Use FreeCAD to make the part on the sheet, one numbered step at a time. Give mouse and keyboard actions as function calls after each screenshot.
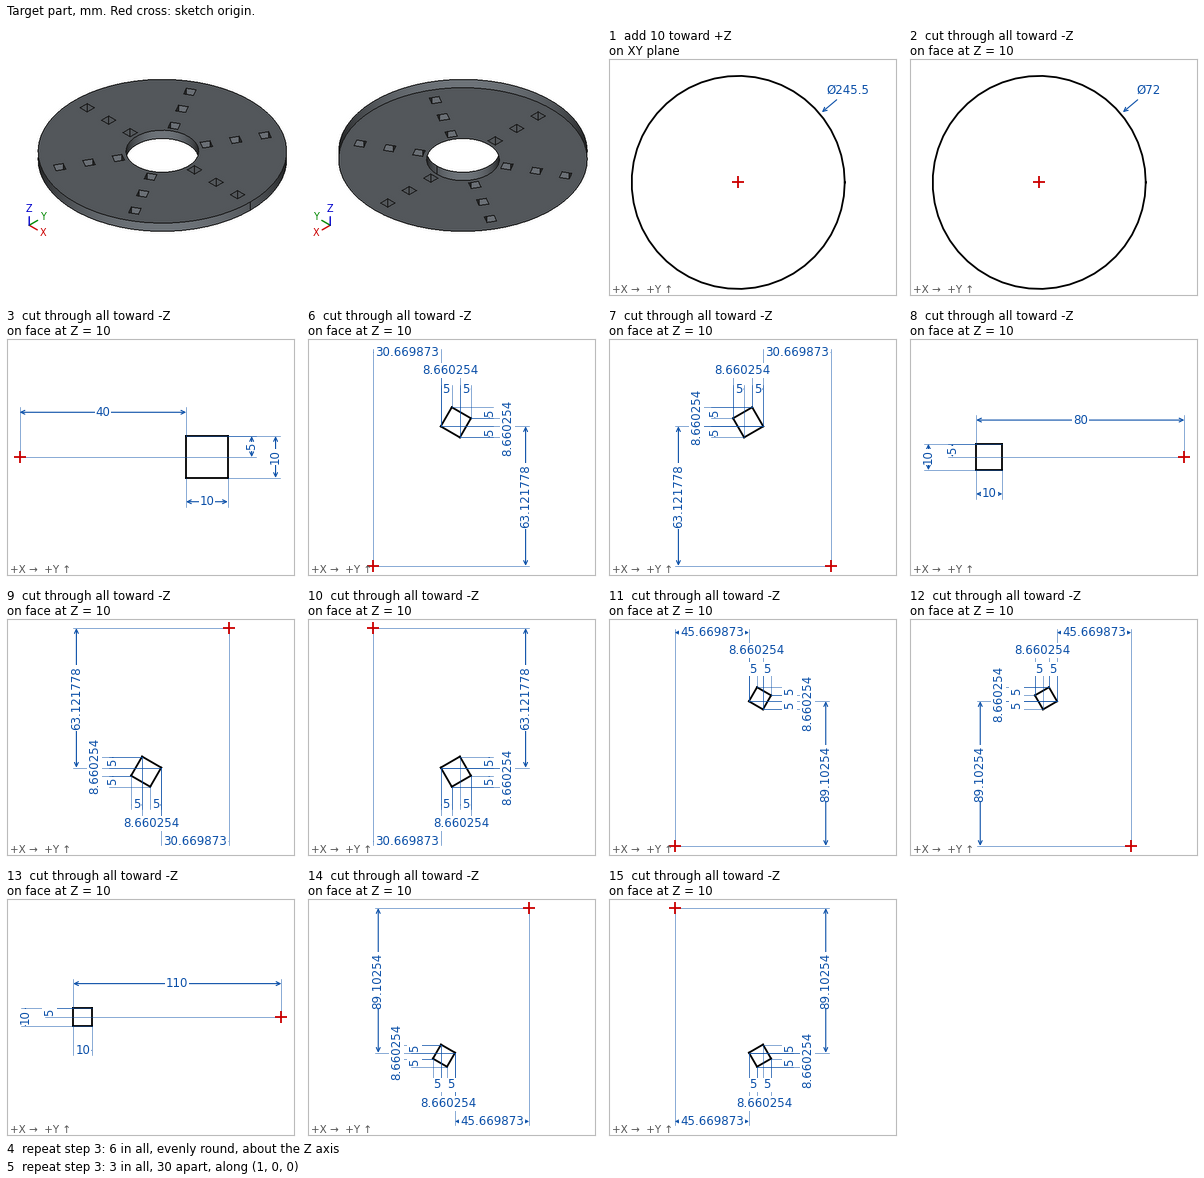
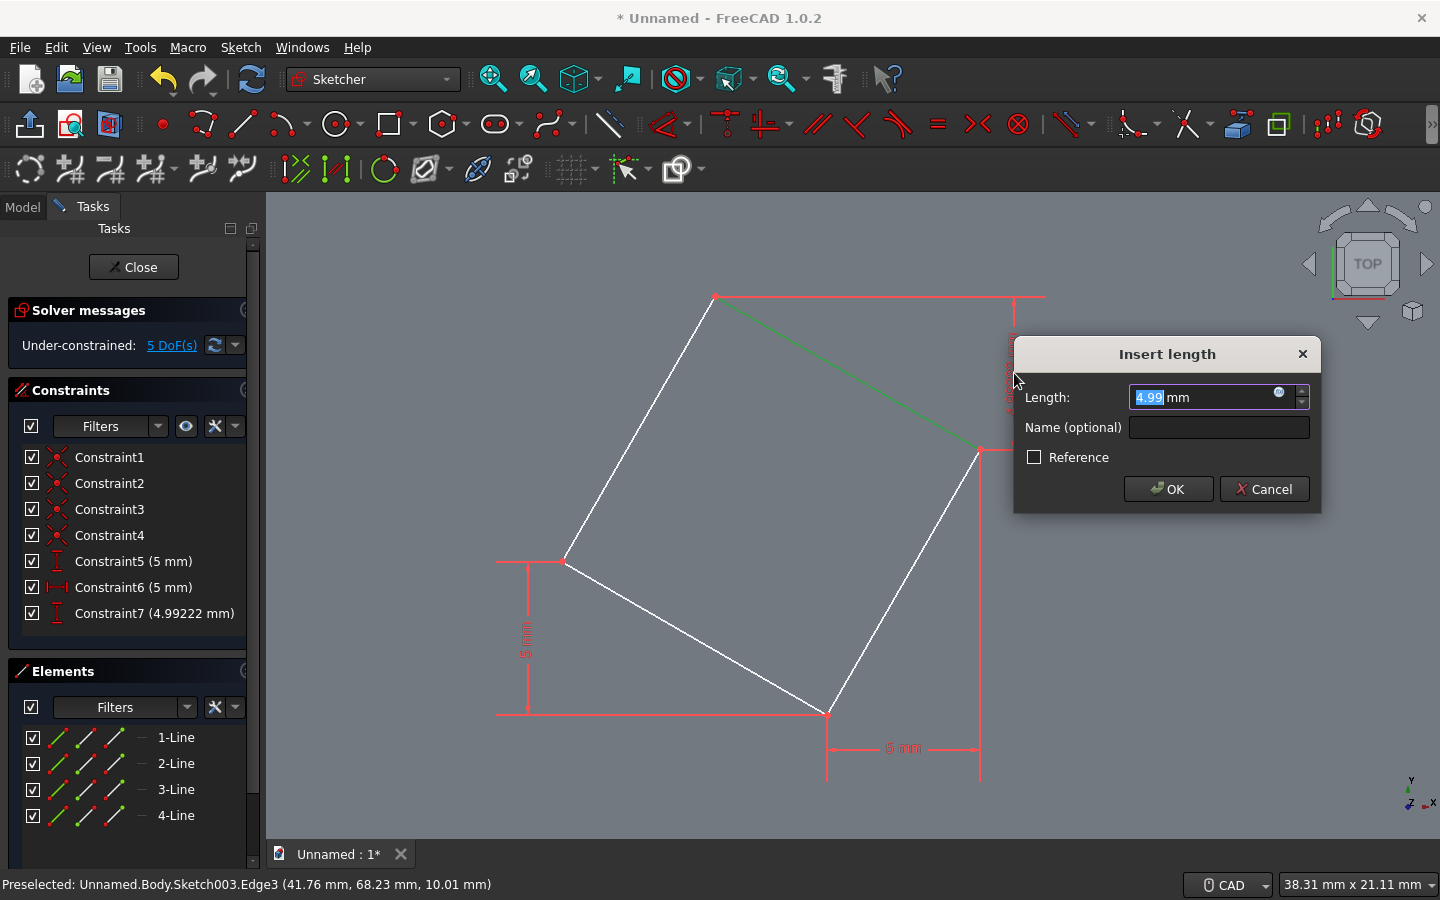
text(5)
key(Return)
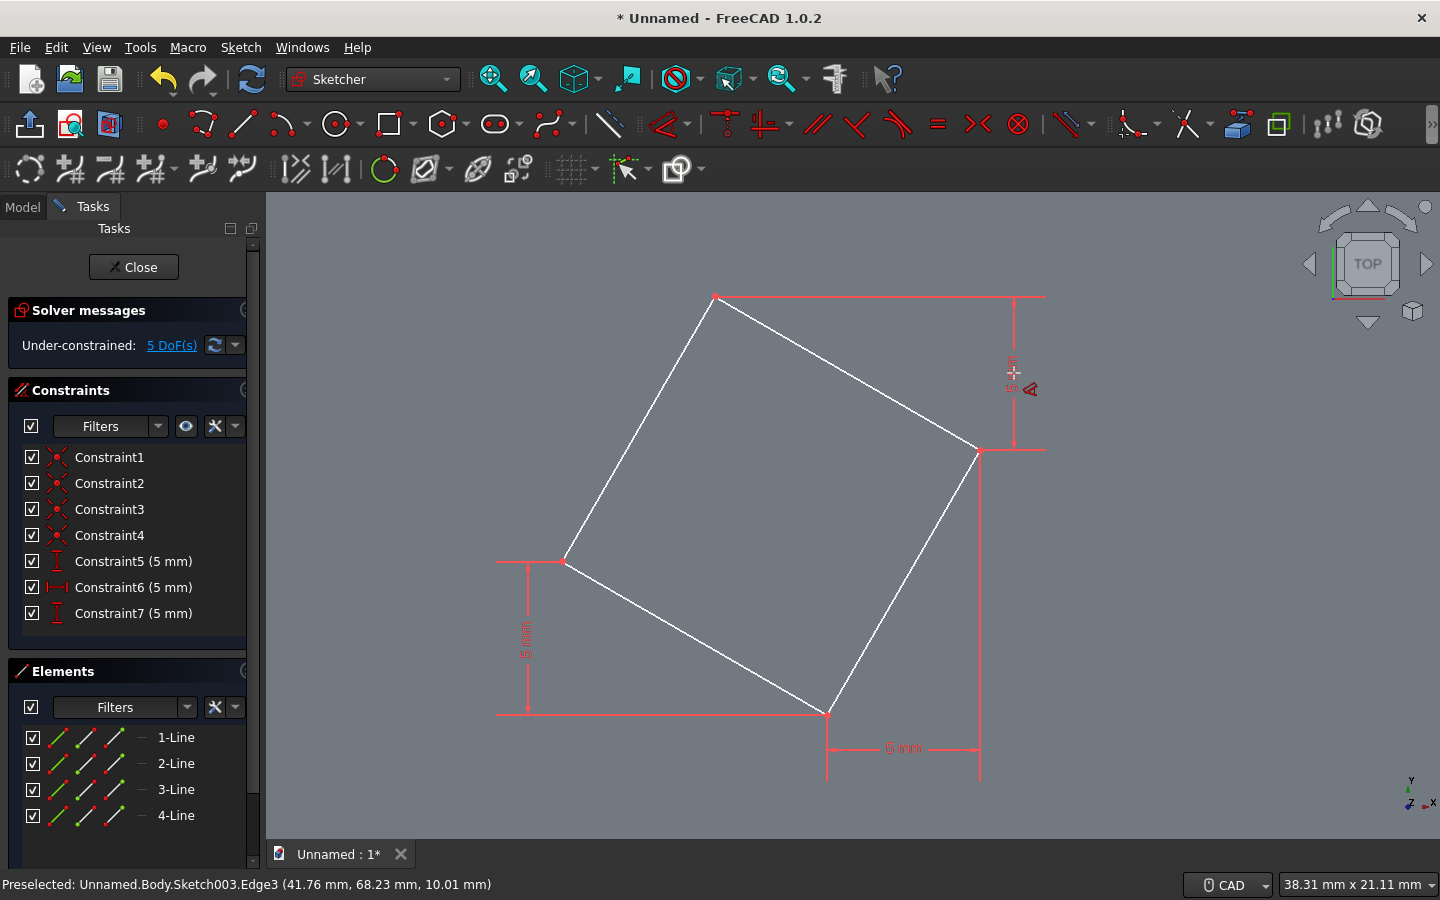
click(669, 376)
click(639, 263)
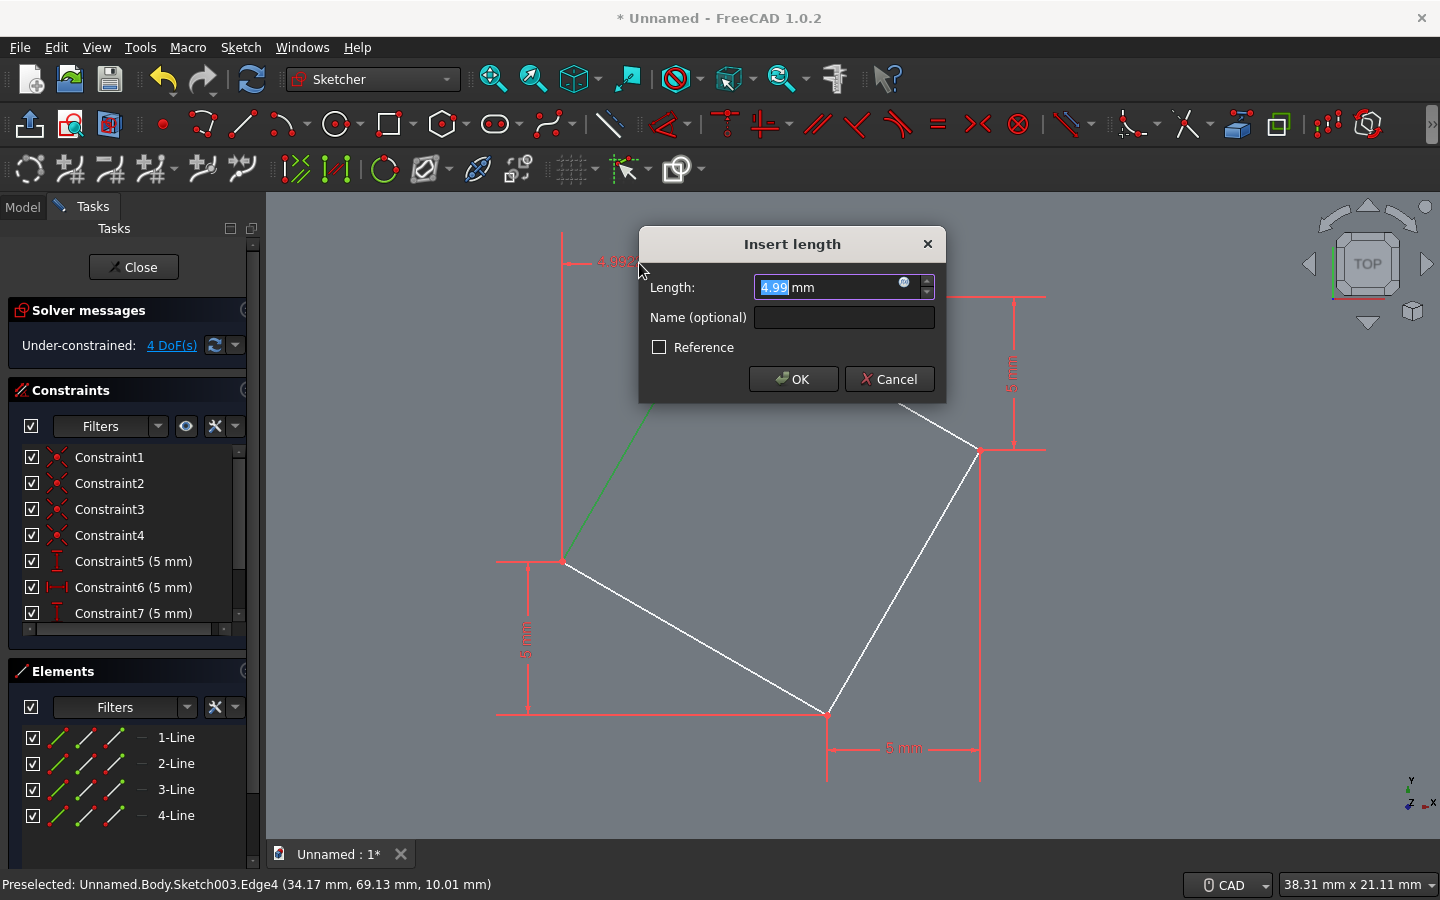
text(5)
key(Return)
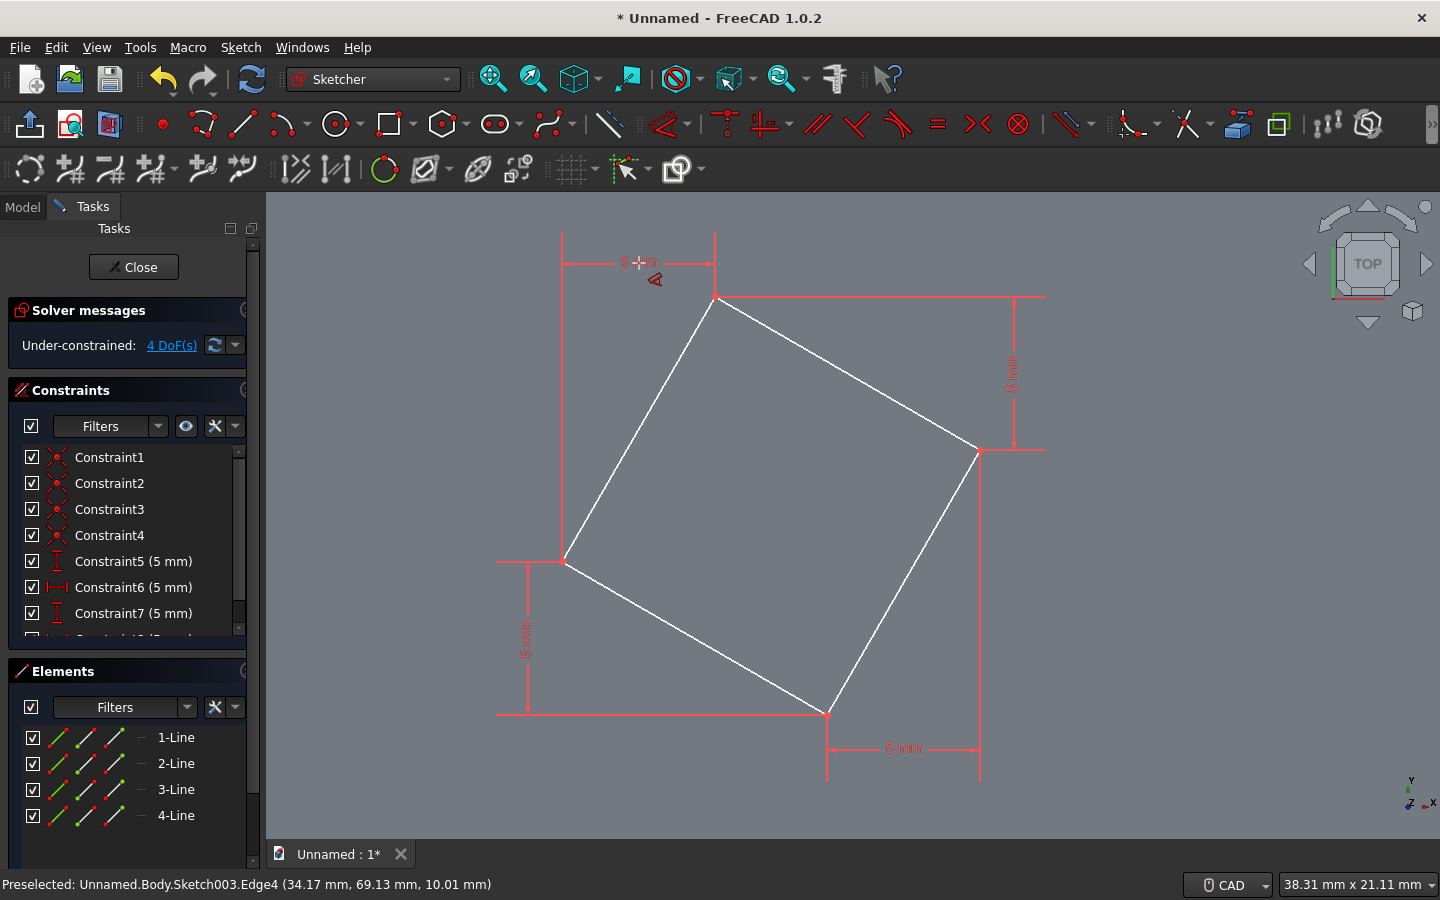
click(642, 608)
click(695, 749)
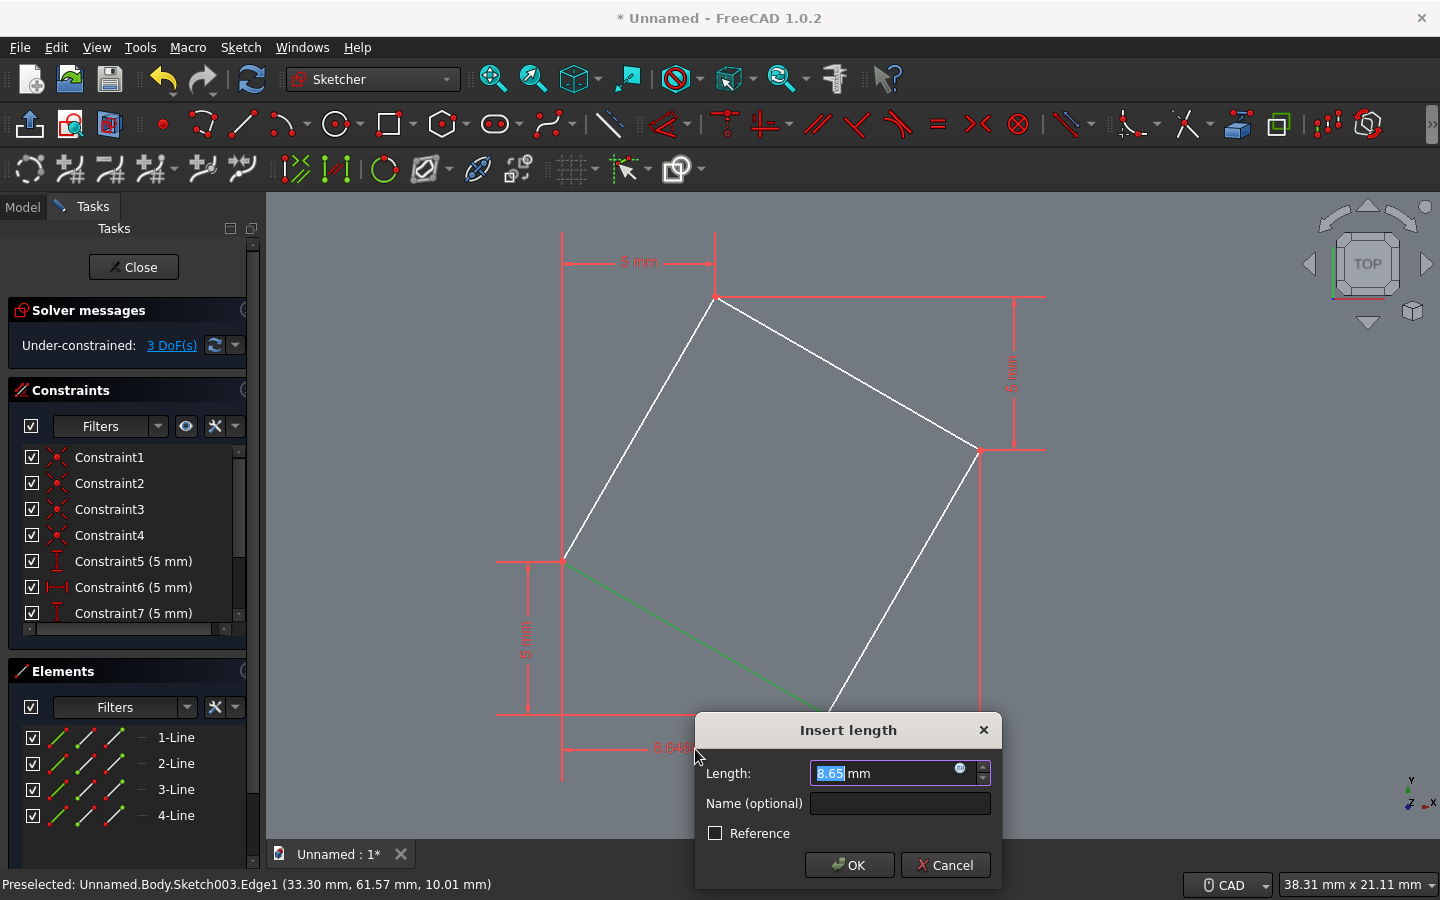
text(8.660254)
key(Return)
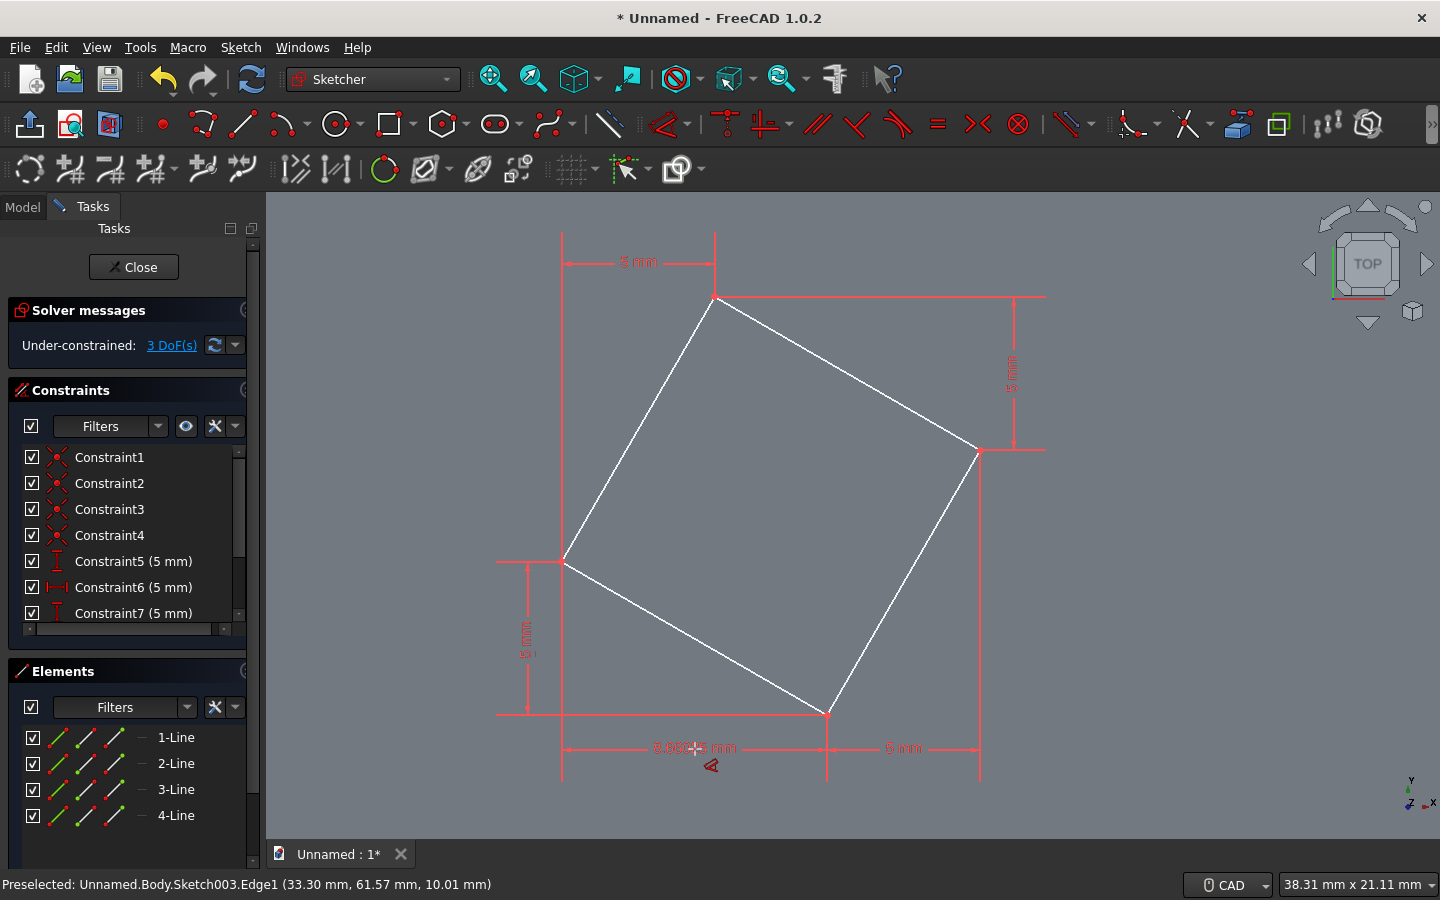
click(873, 636)
click(1014, 583)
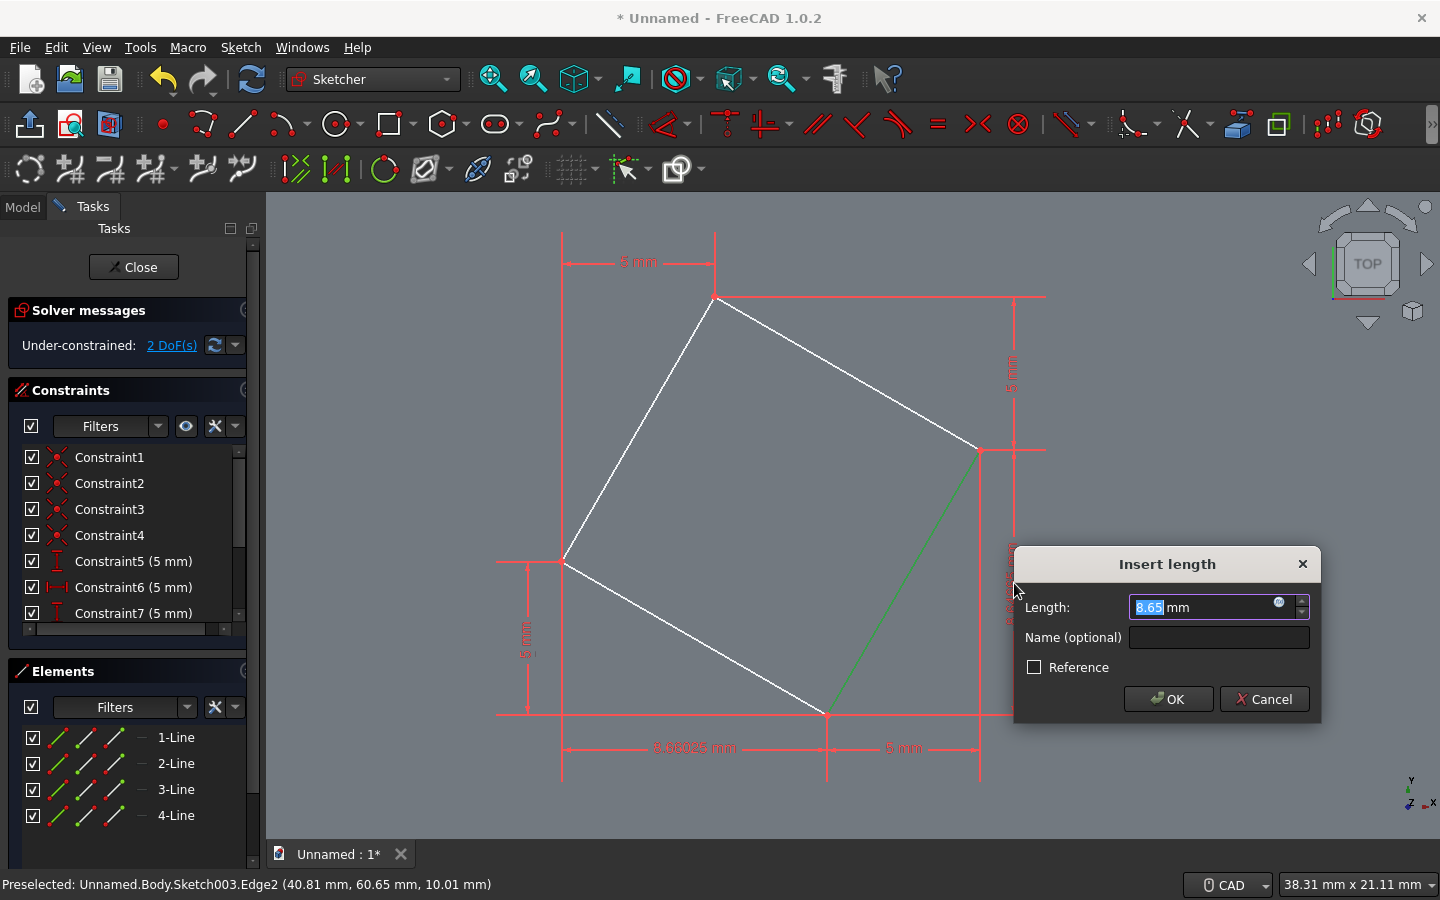
text(8.660254)
key(Return)